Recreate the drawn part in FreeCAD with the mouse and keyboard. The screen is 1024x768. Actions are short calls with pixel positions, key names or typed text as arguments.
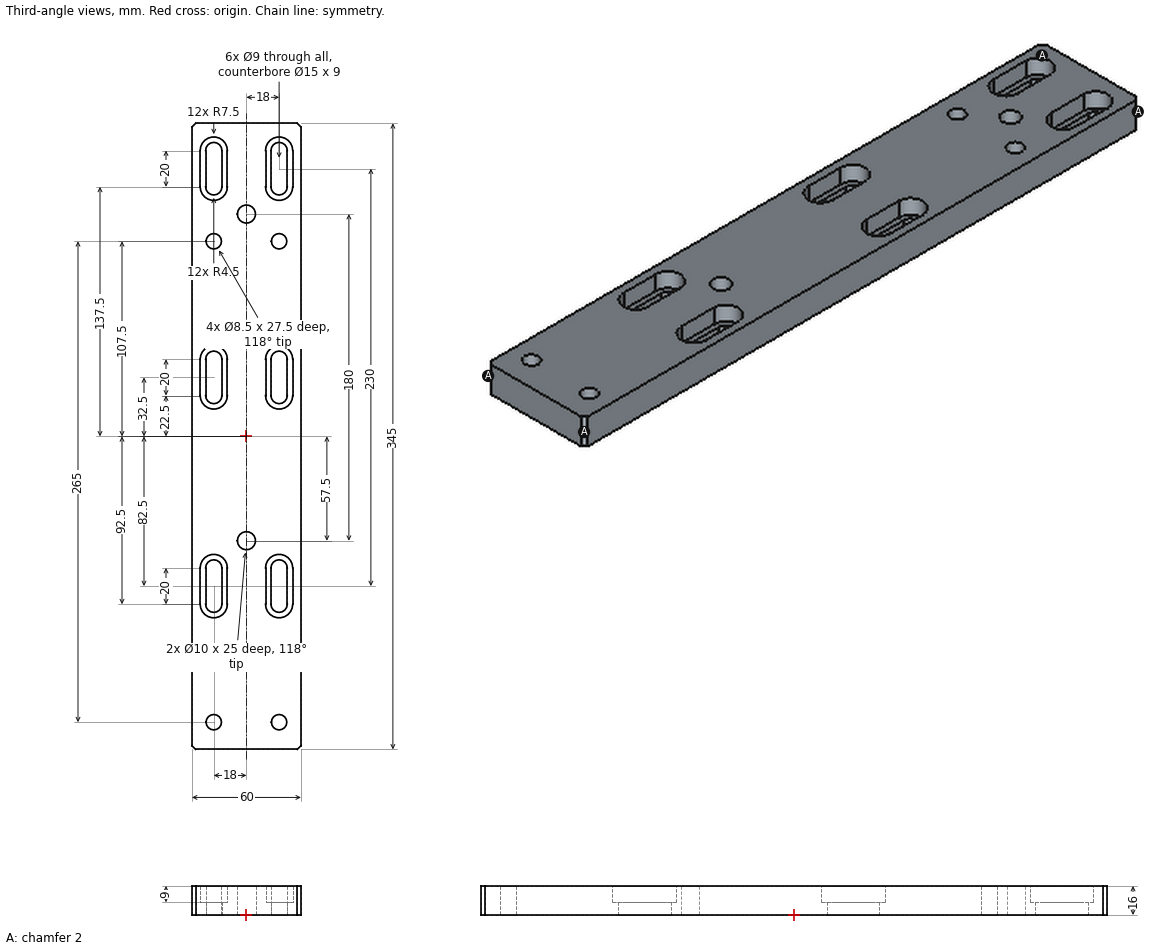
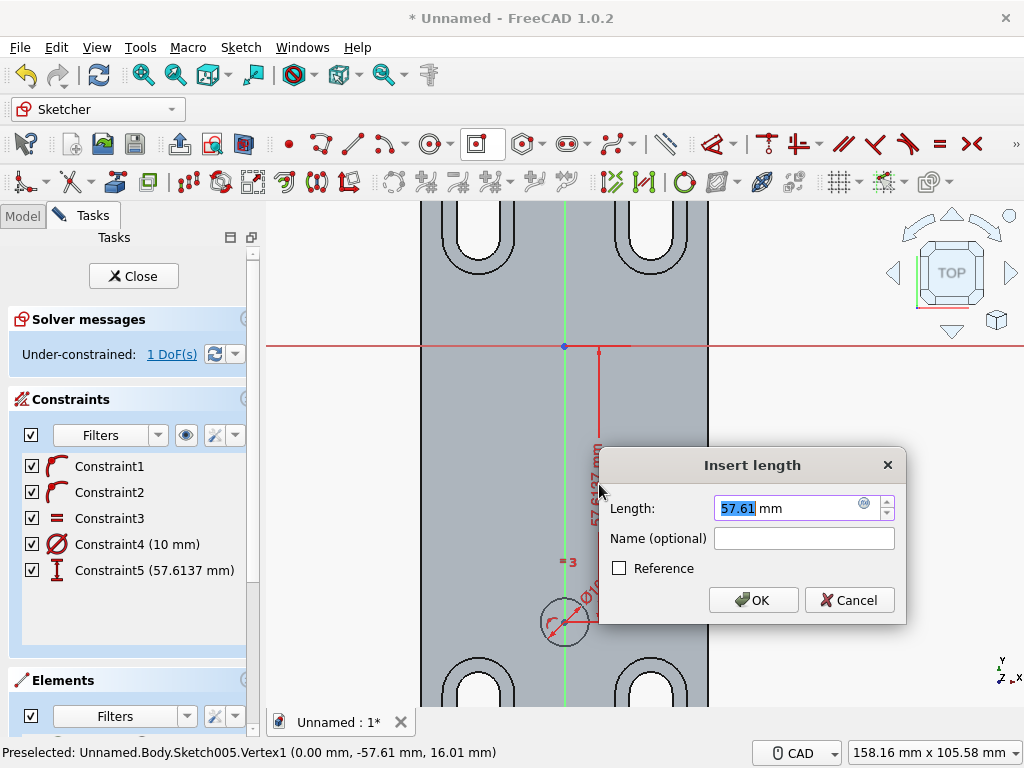
text(57.5)
key(Return)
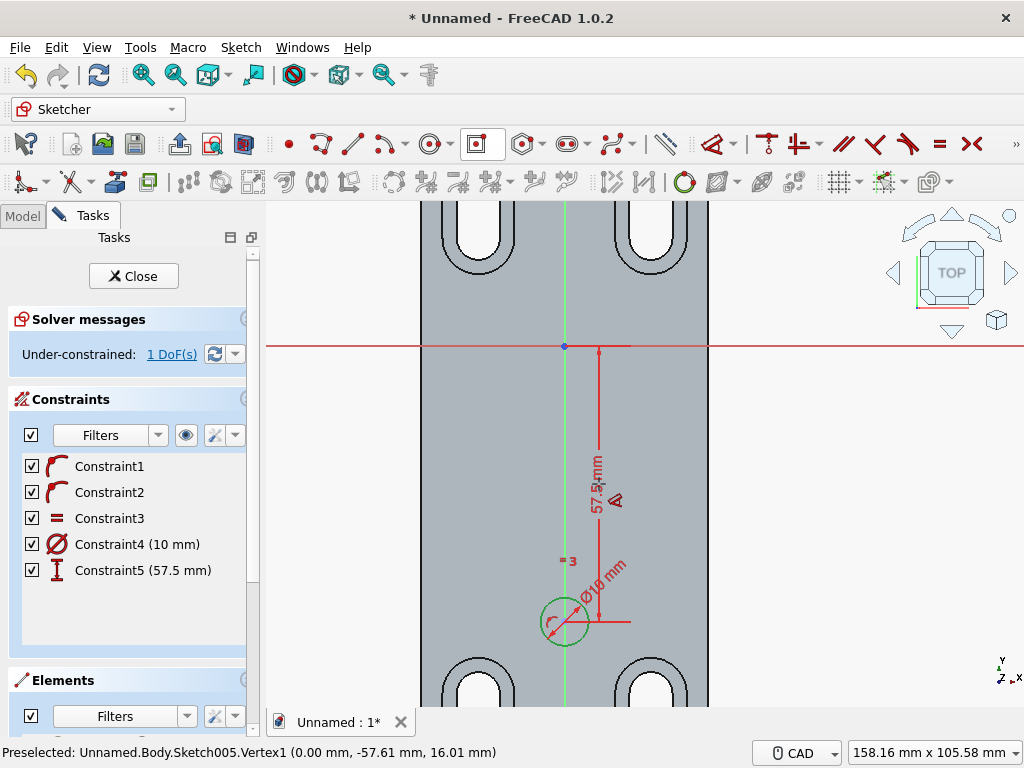
click(565, 622)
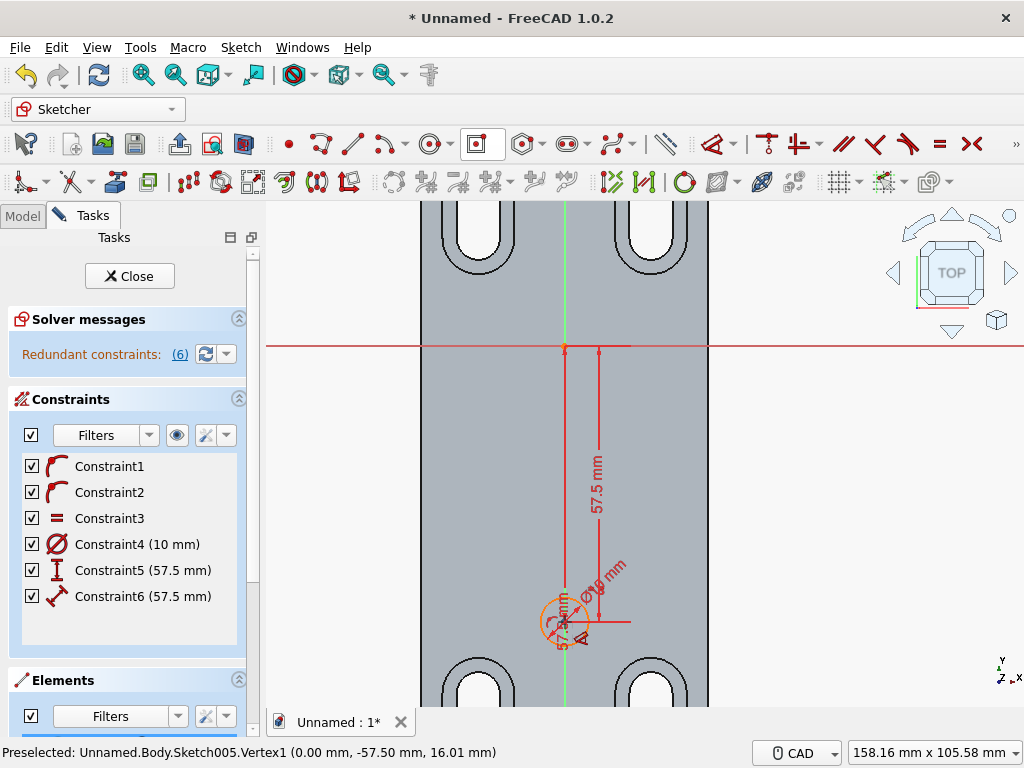
scroll(583, 607, down, 5)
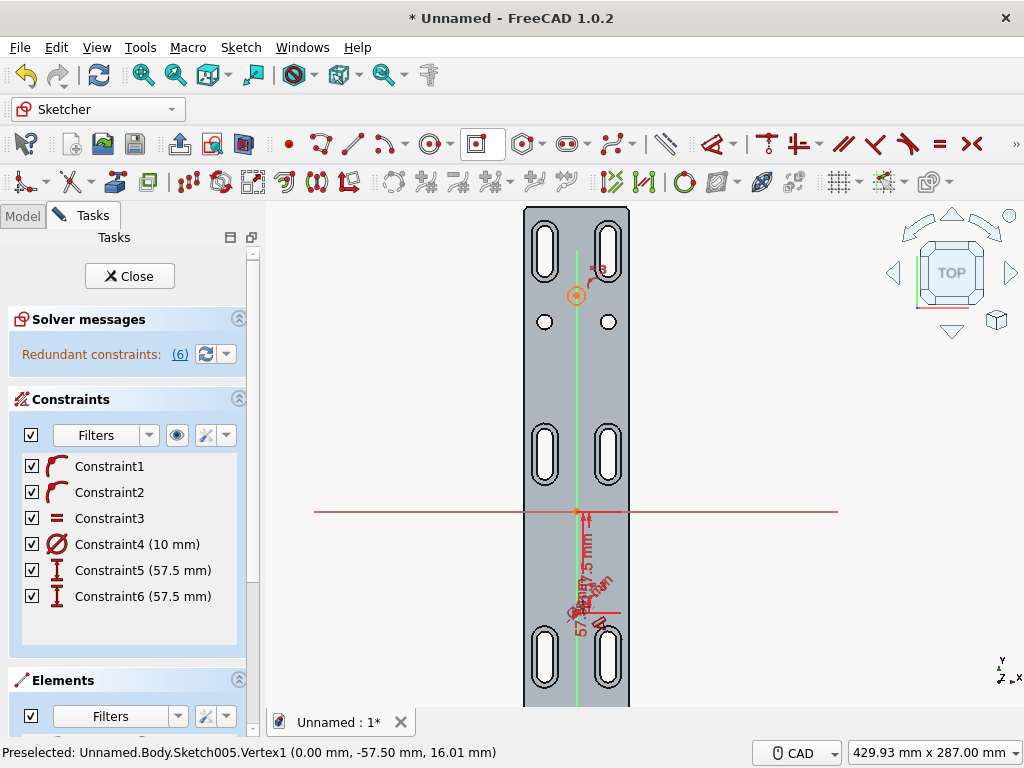
click(577, 296)
click(611, 454)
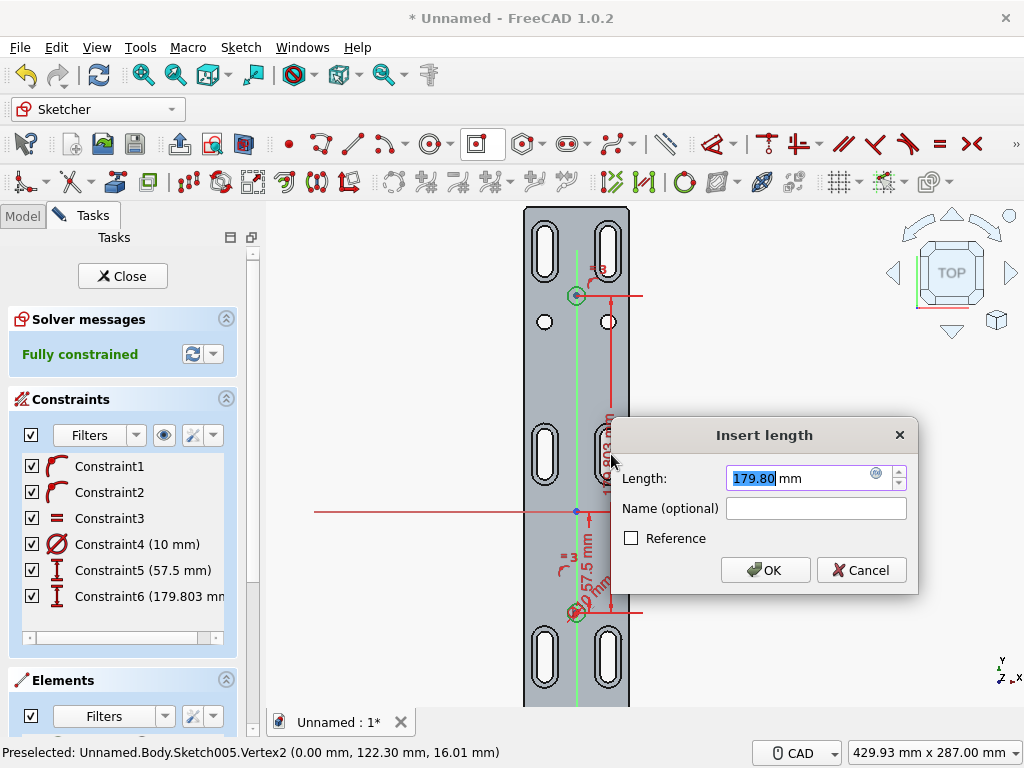
text(180)
key(Return)
key(Escape)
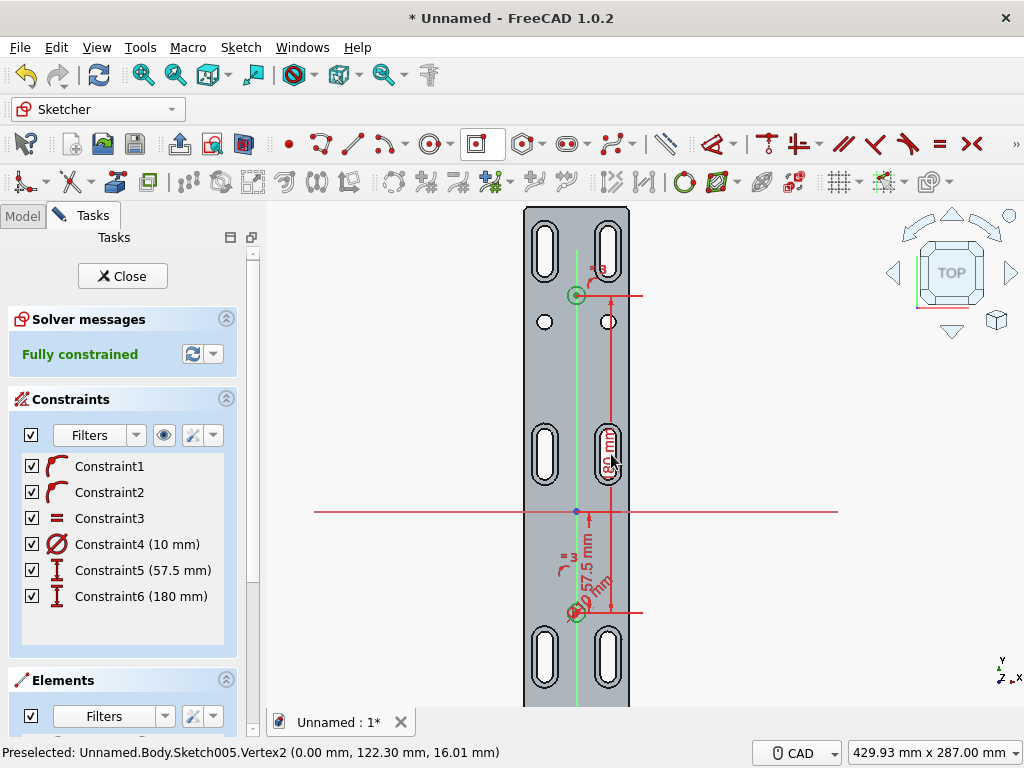
click(123, 276)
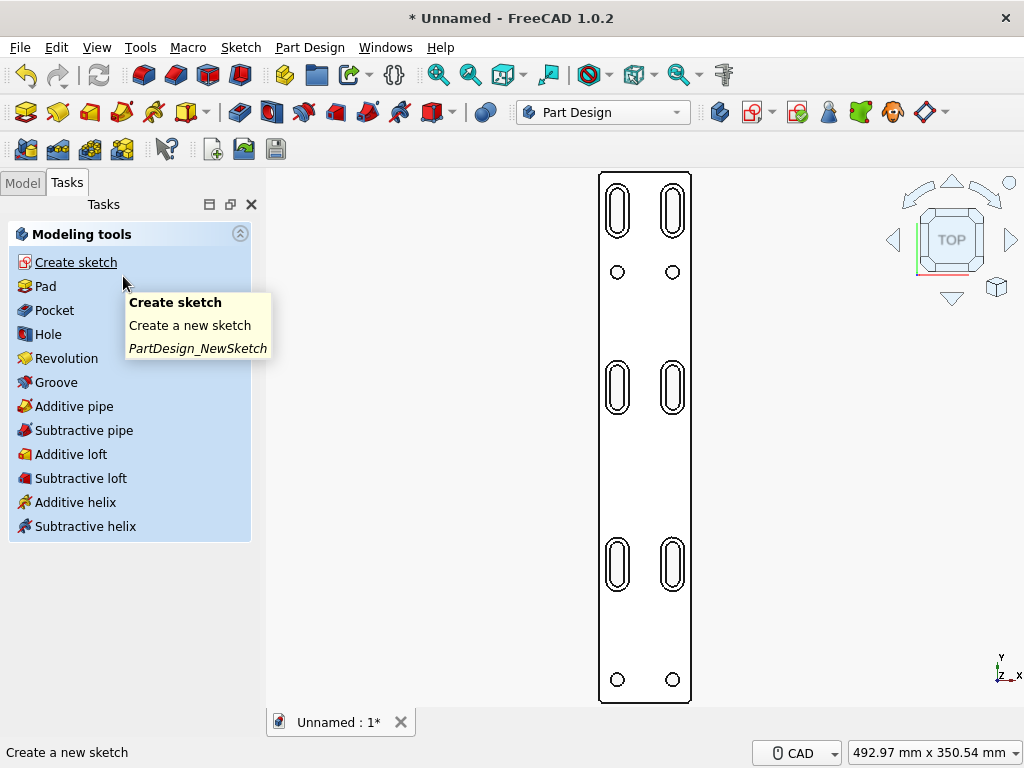
click(272, 112)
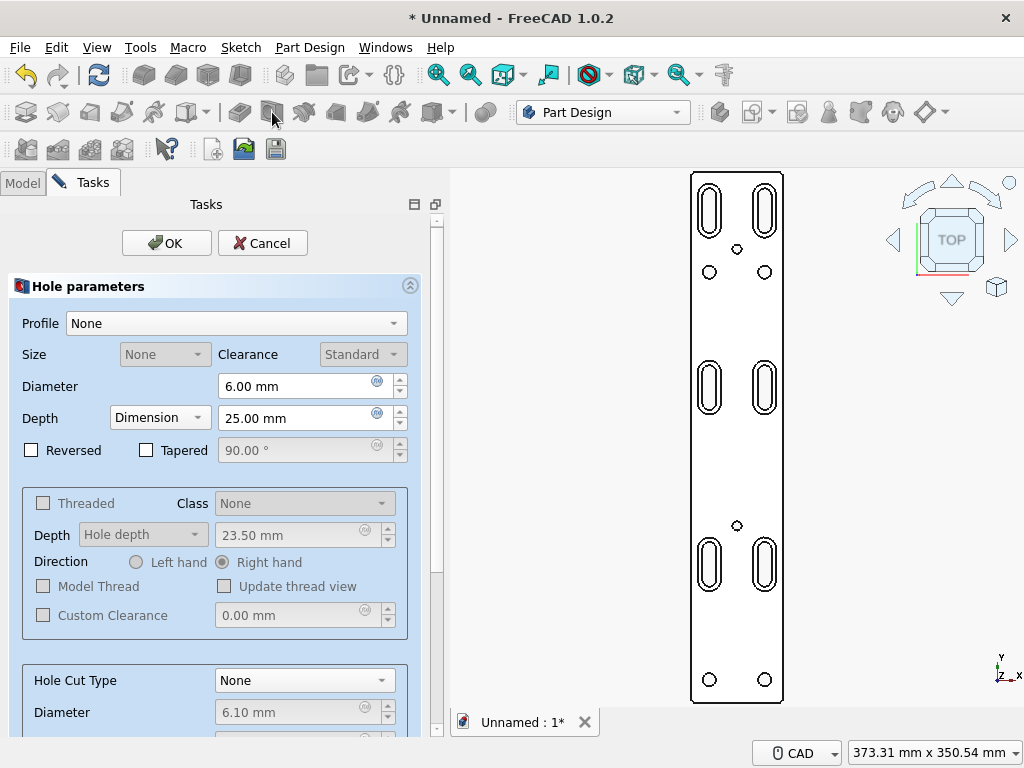
triple_click(305, 386)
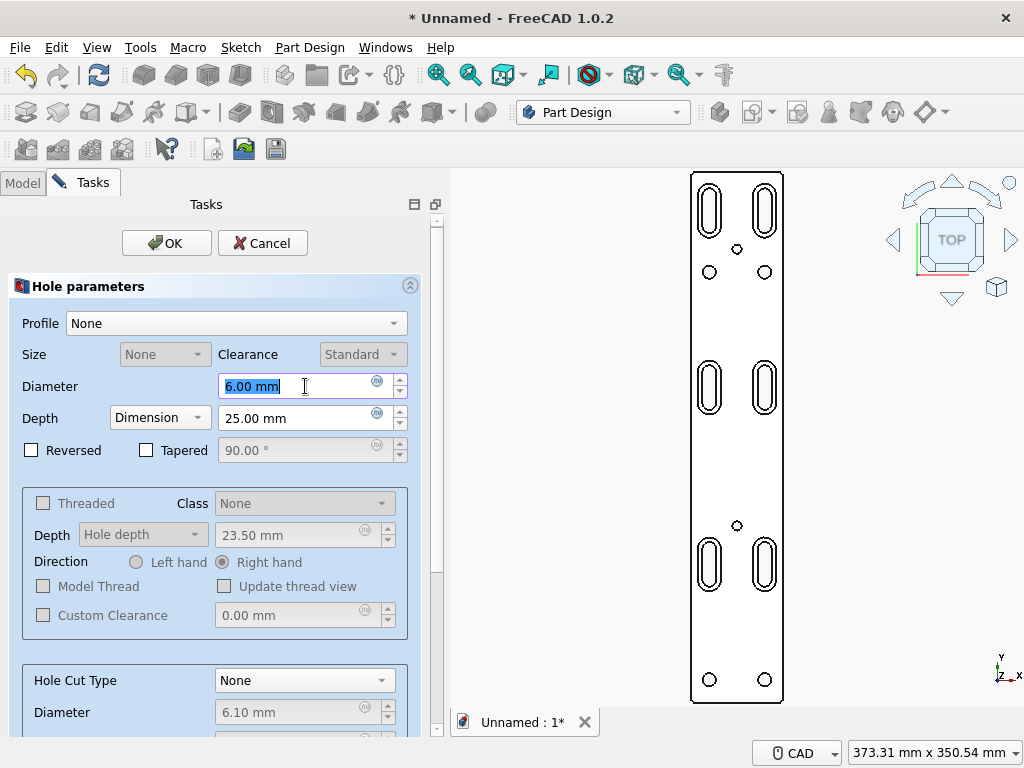
text(10)
key(Tab)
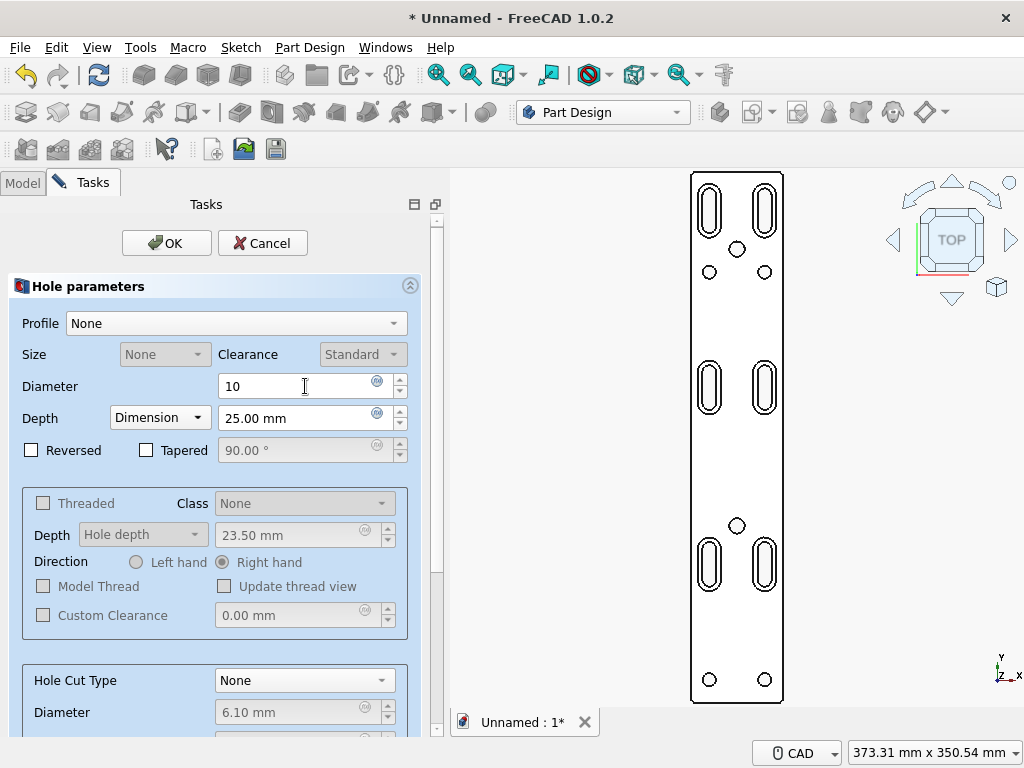
triple_click(305, 418)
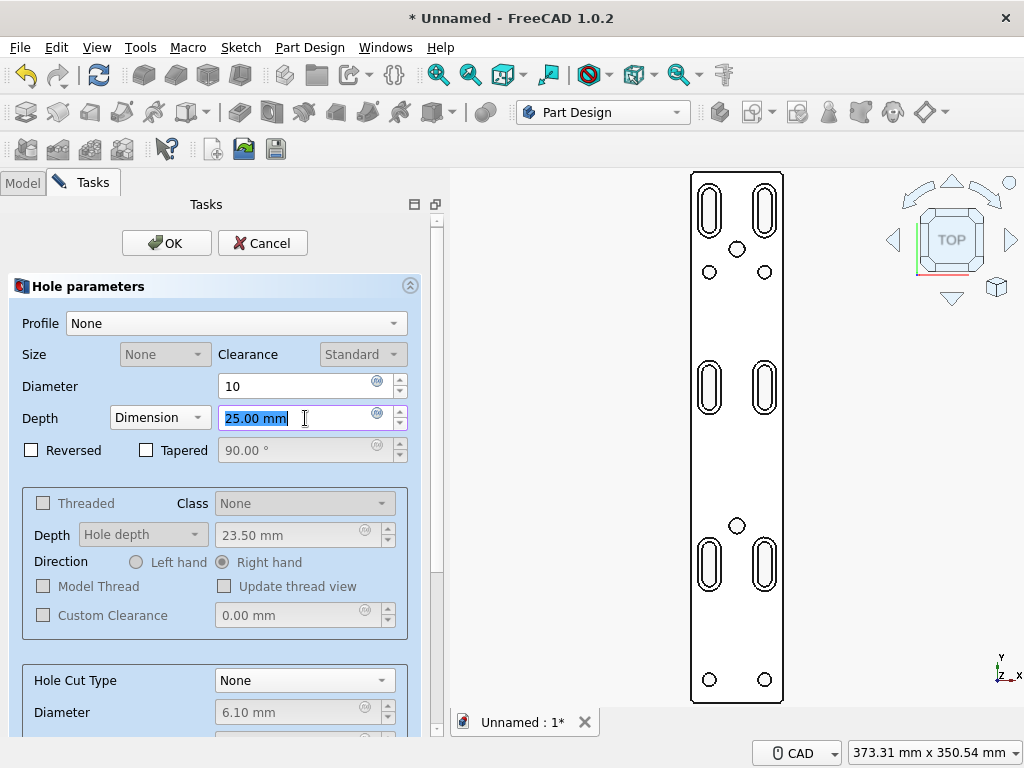
text(25)
key(Tab)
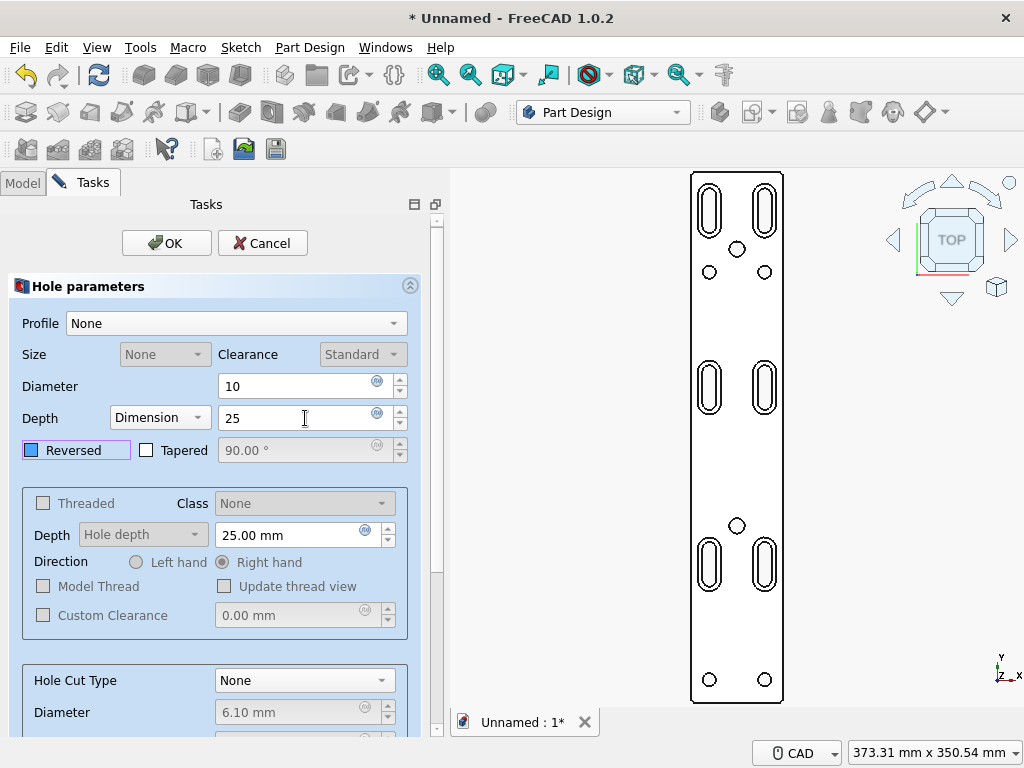
click(167, 243)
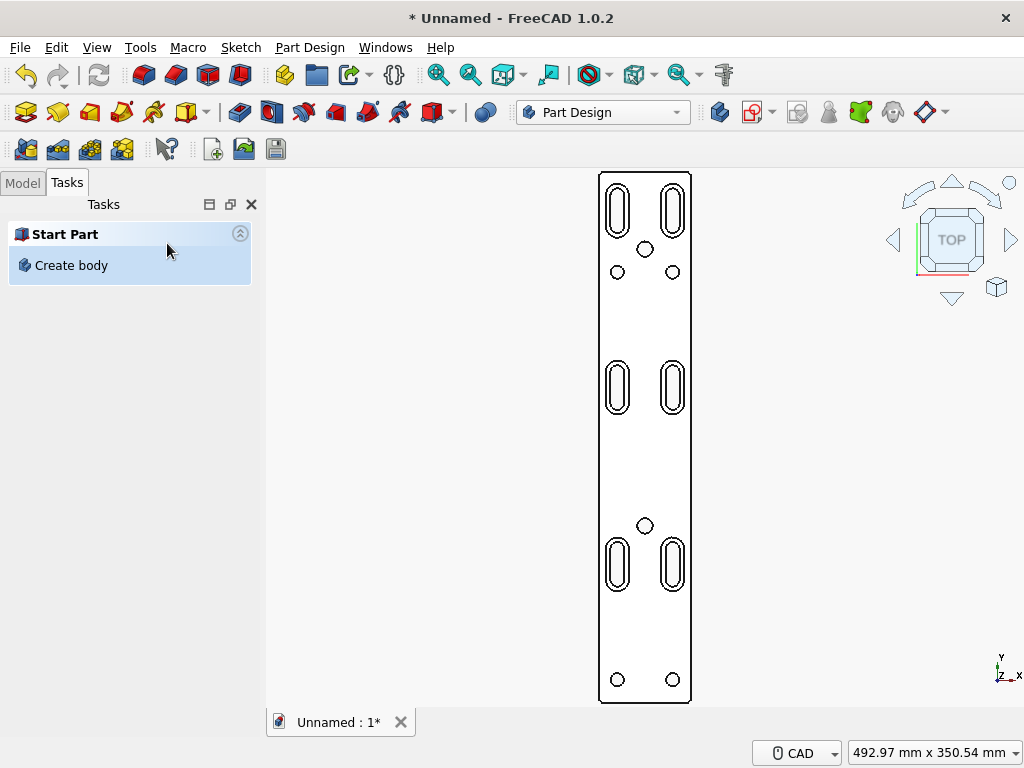
key(0)